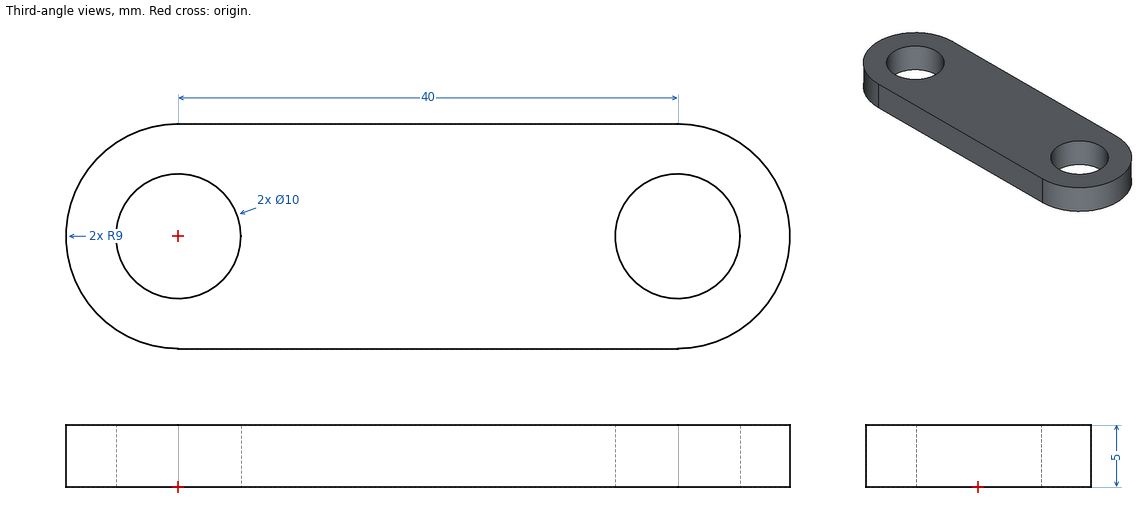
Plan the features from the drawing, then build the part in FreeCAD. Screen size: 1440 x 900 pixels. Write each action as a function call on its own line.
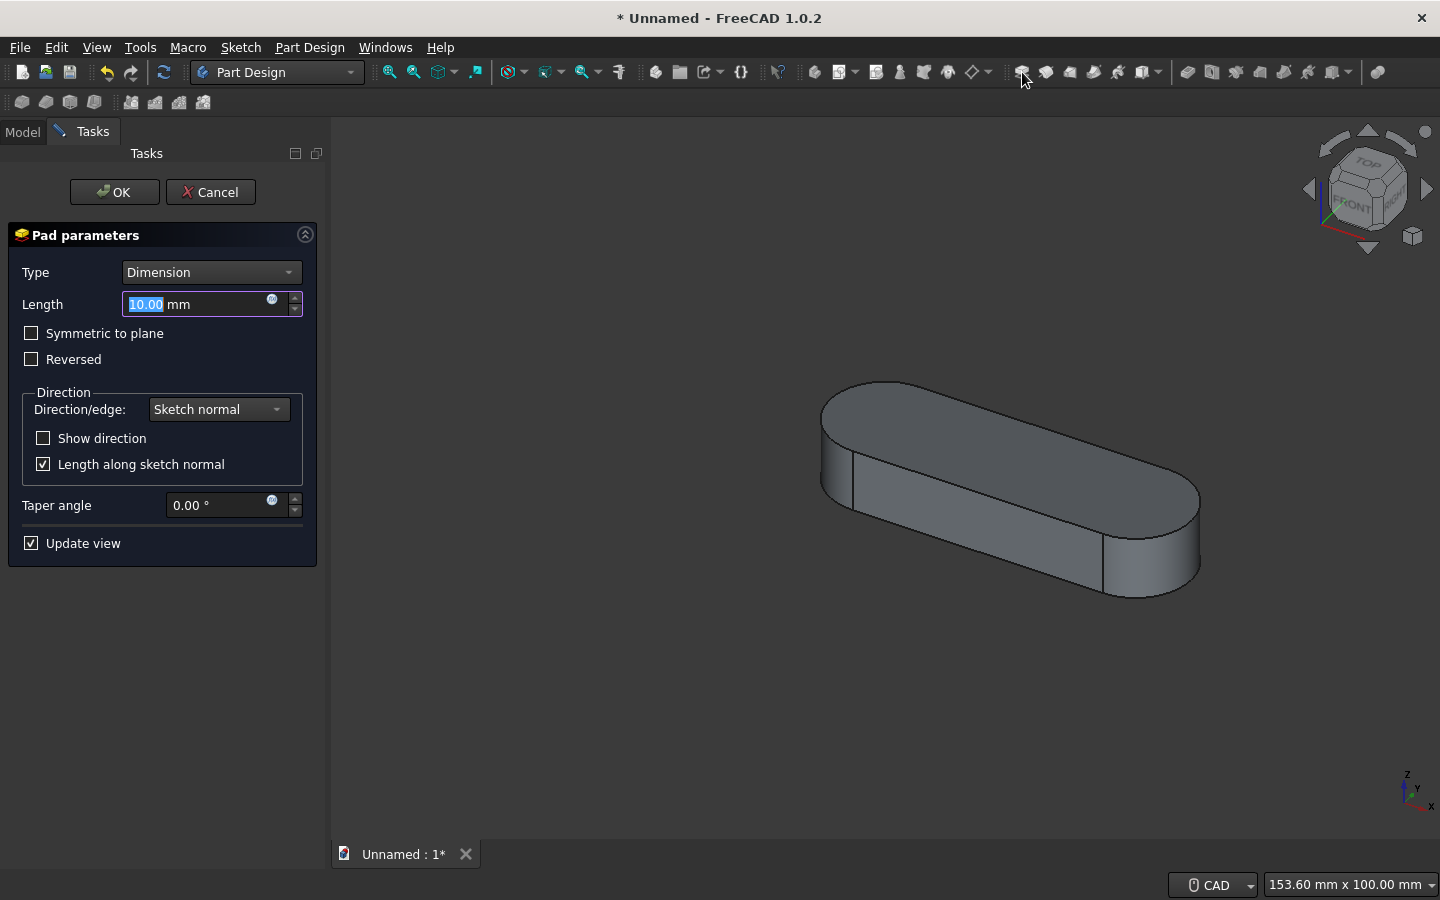
text(5)
key(Tab)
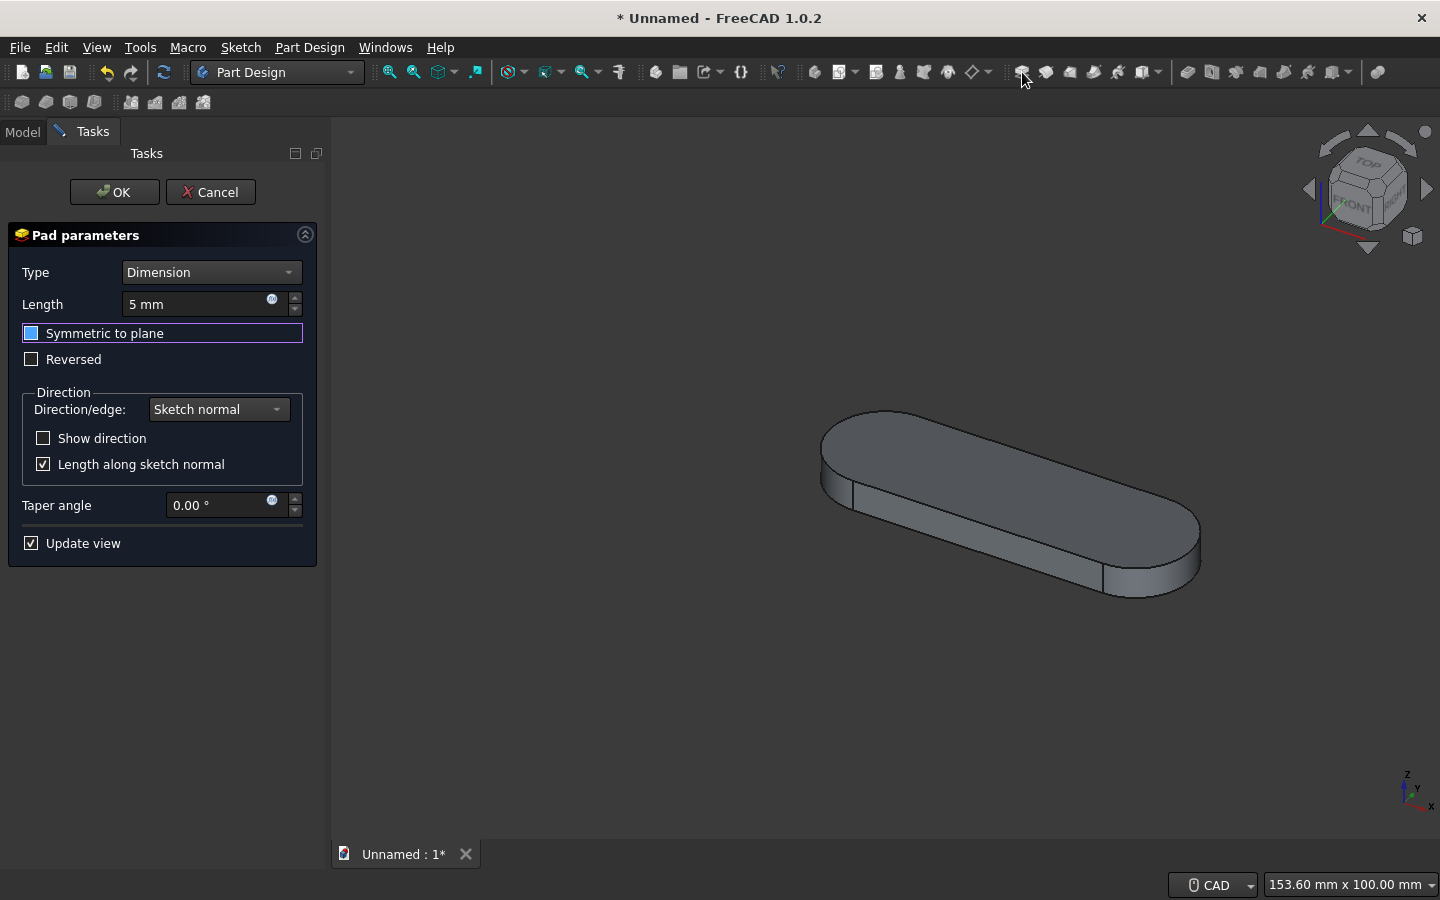
click(115, 192)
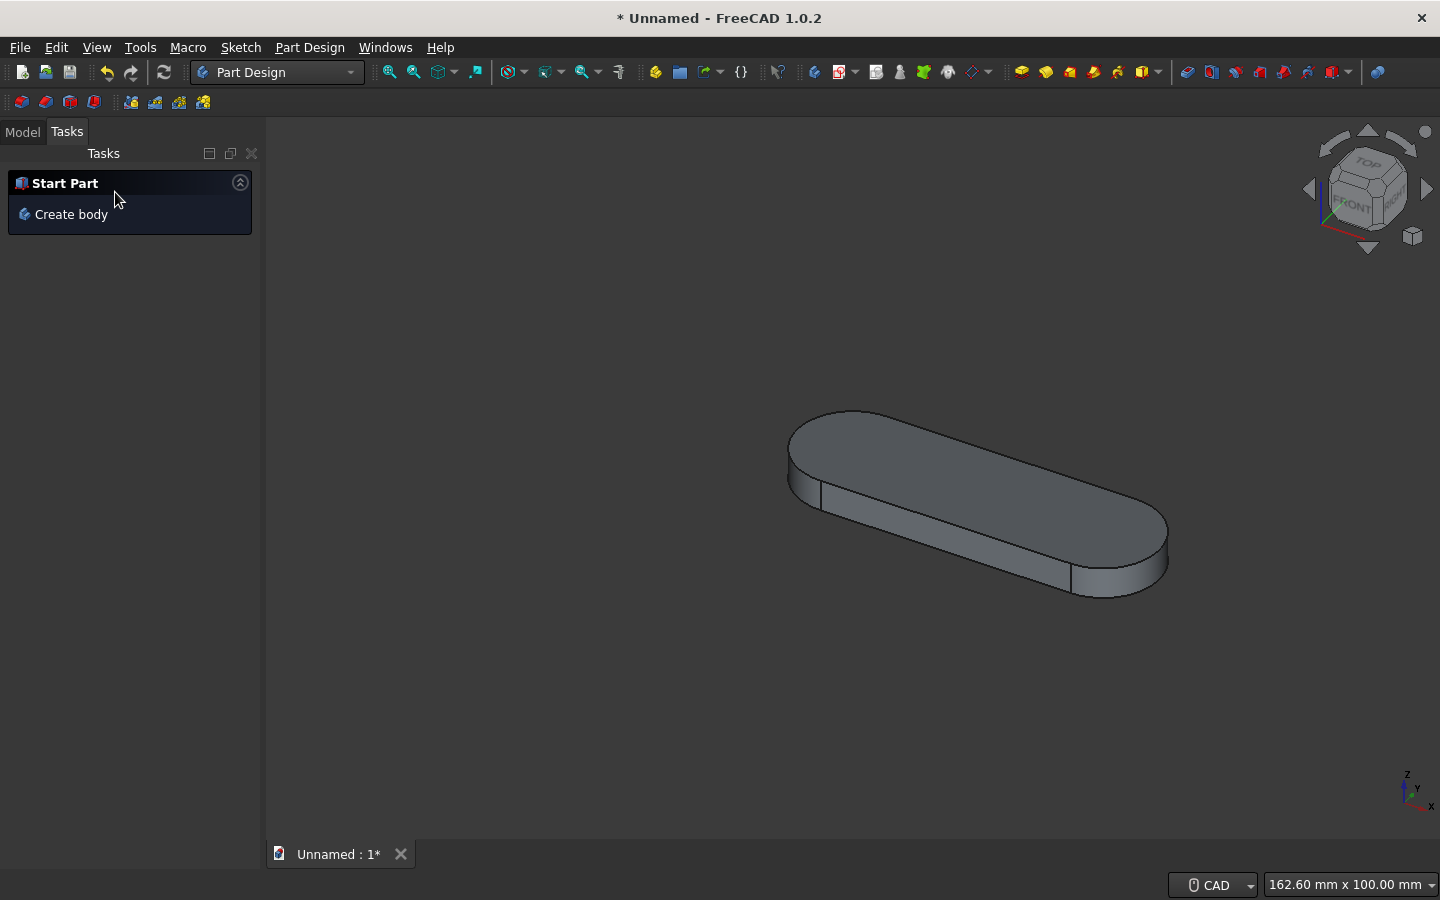
click(390, 72)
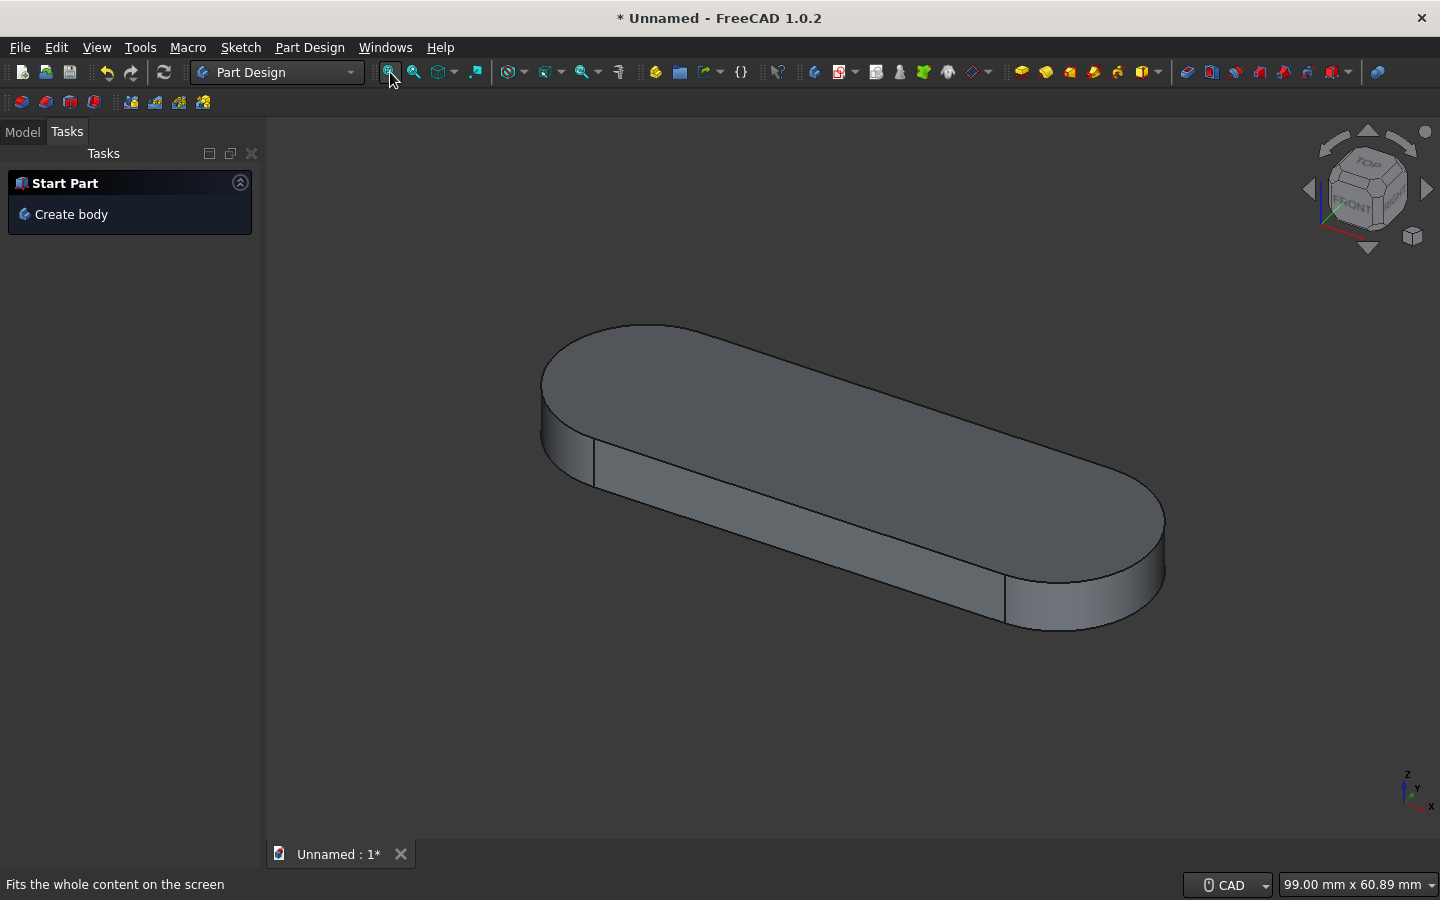
click(1023, 509)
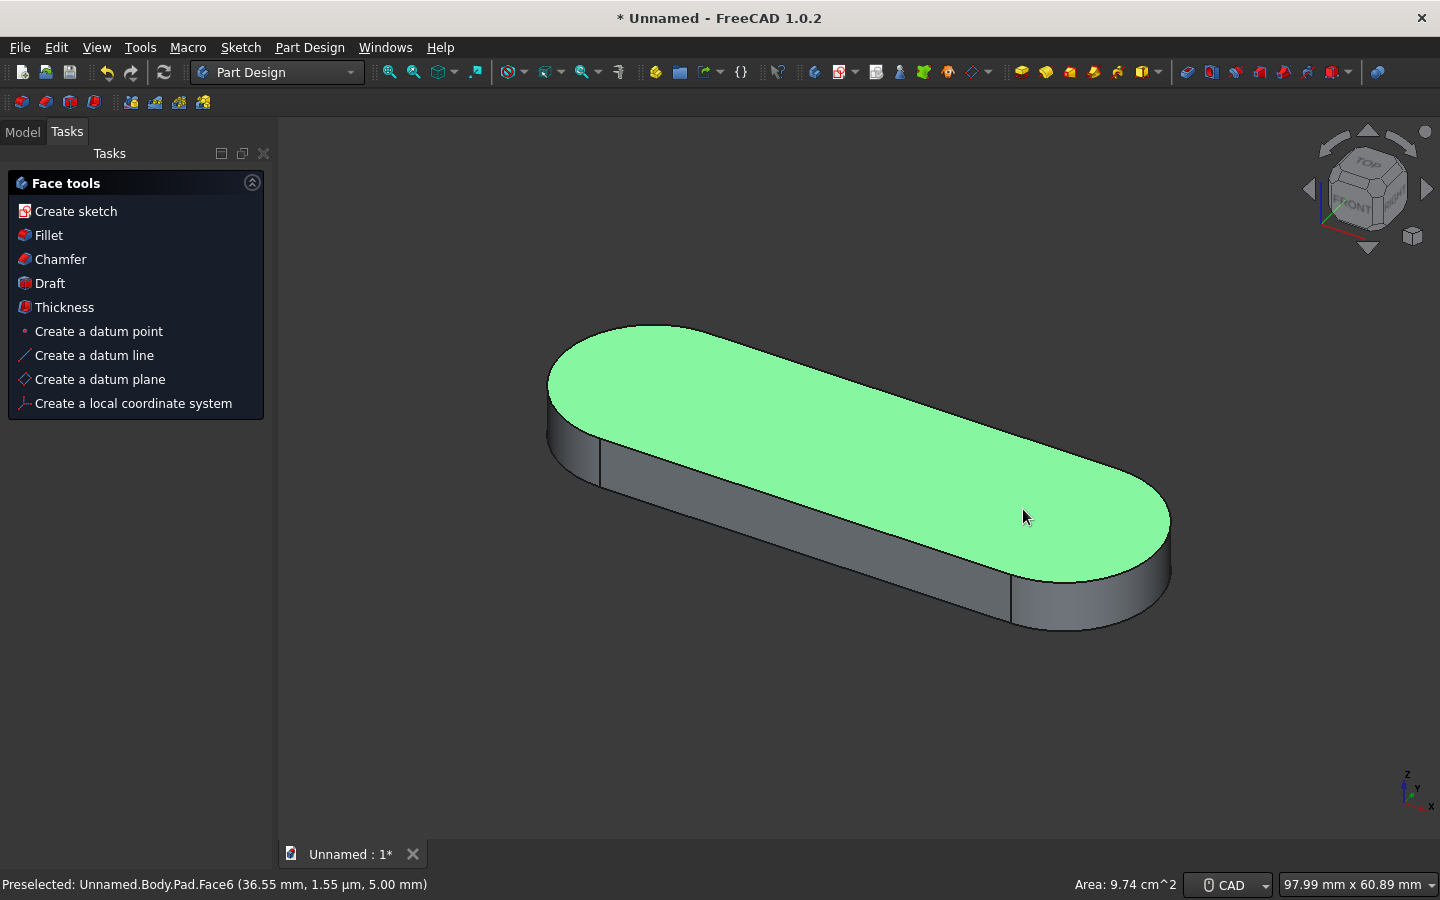
click(840, 72)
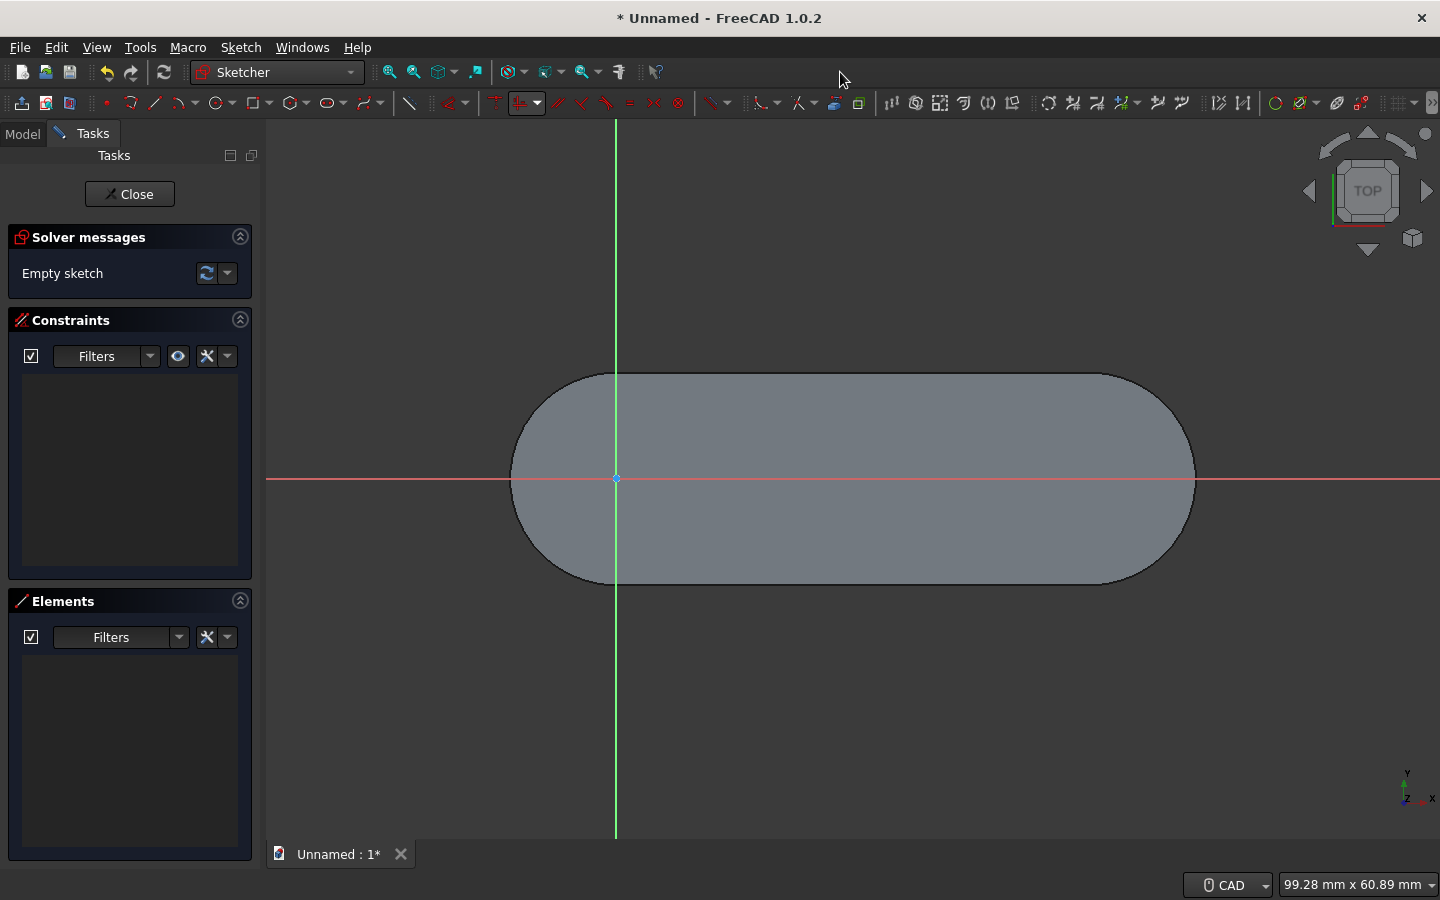
click(216, 104)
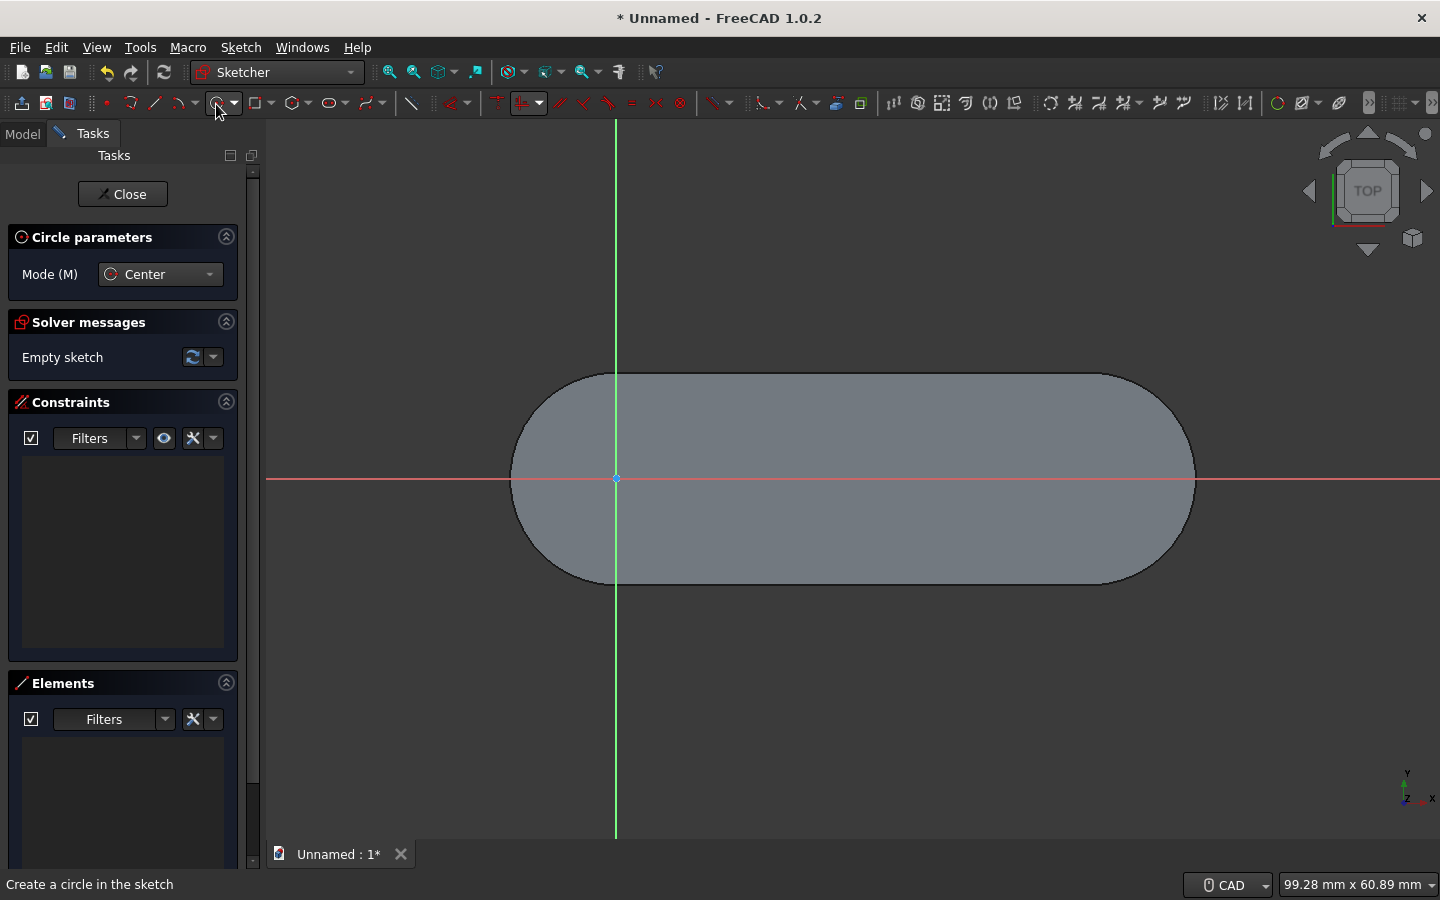
click(616, 479)
click(658, 437)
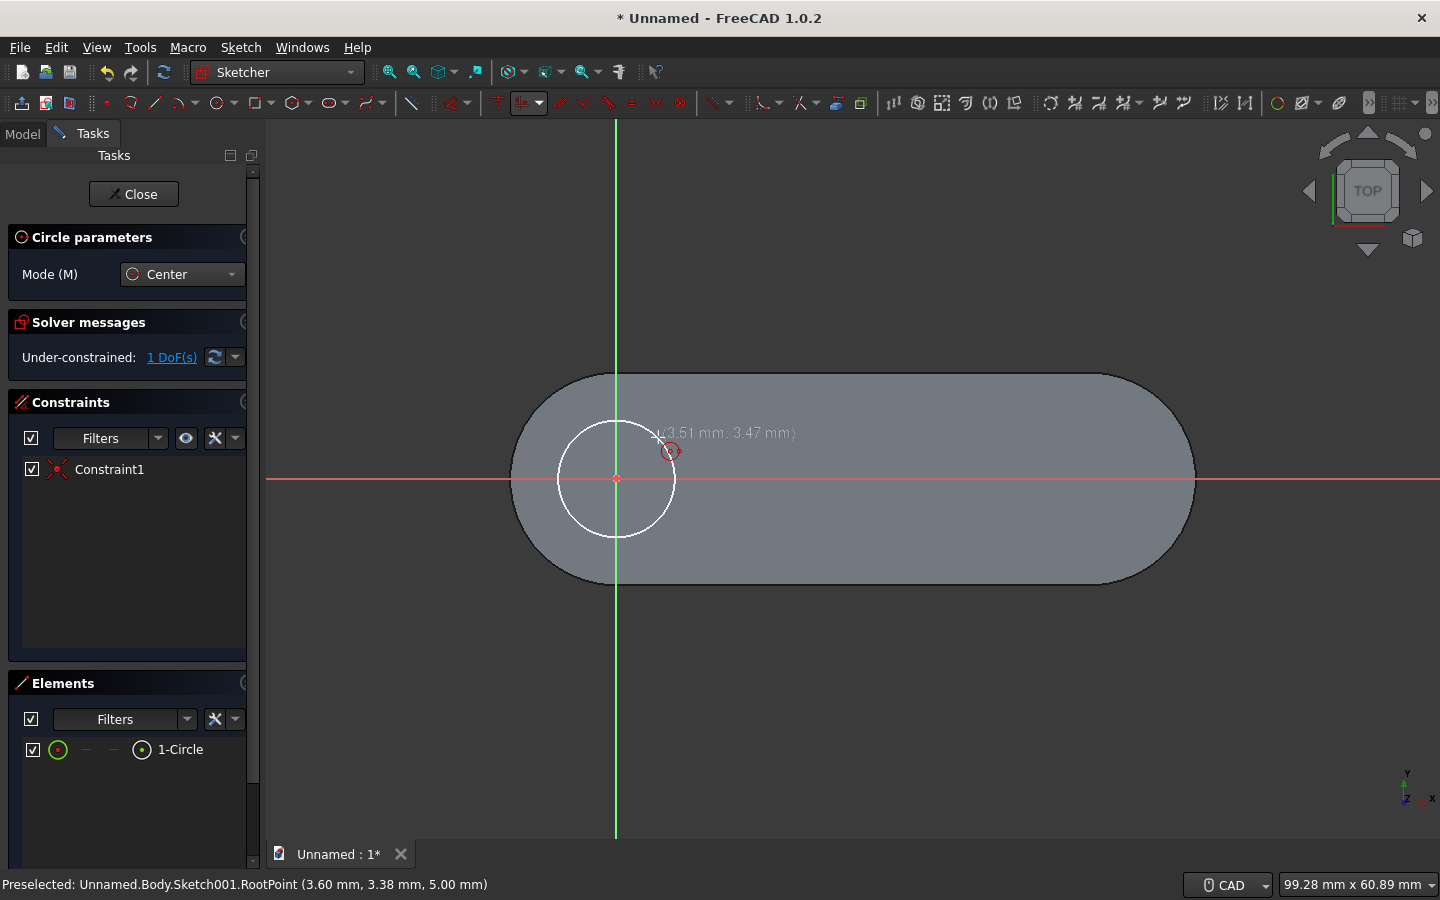
click(1090, 479)
click(1131, 437)
key(Escape)